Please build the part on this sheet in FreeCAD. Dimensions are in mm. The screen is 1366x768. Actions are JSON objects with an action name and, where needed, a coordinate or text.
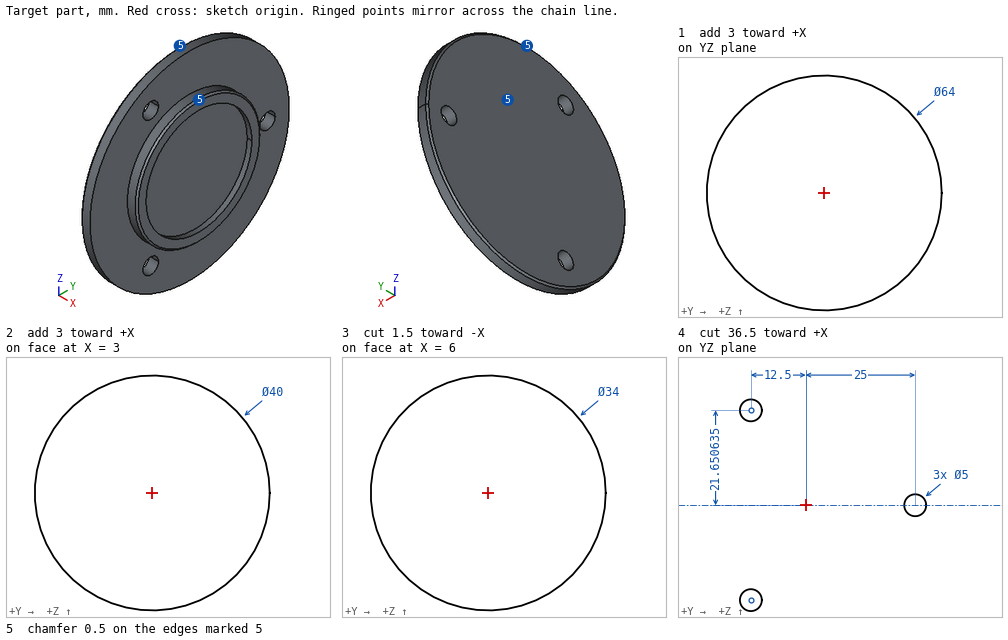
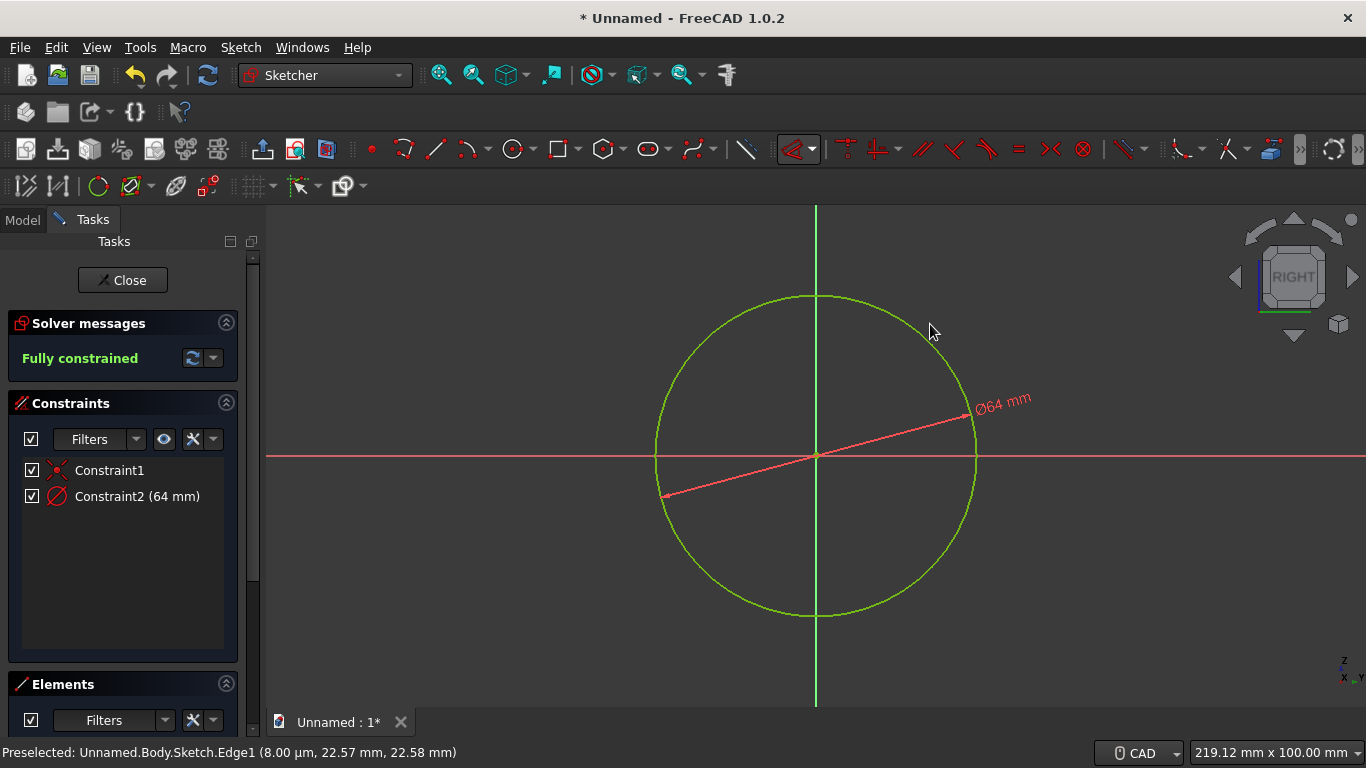
{"action": "left_click", "coordinate": [123, 280]}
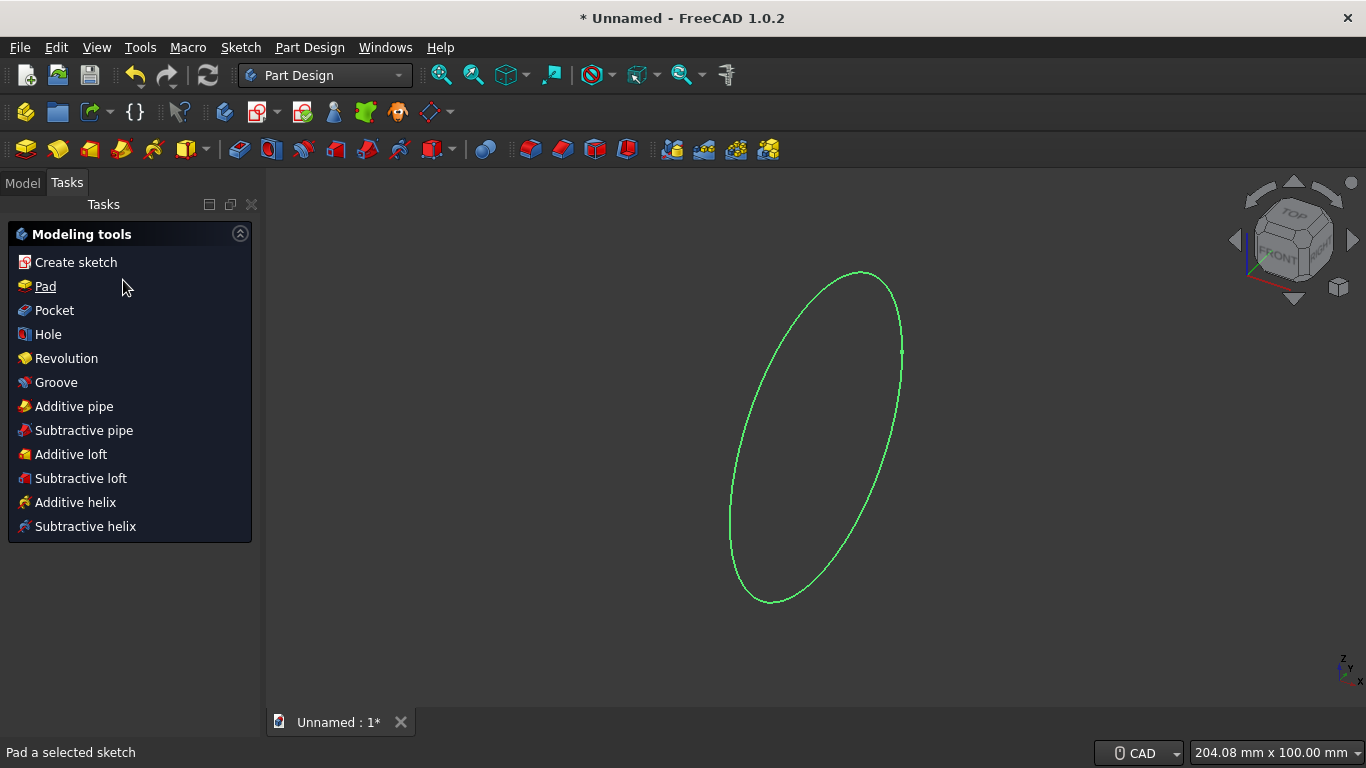
{"action": "left_click", "coordinate": [26, 150]}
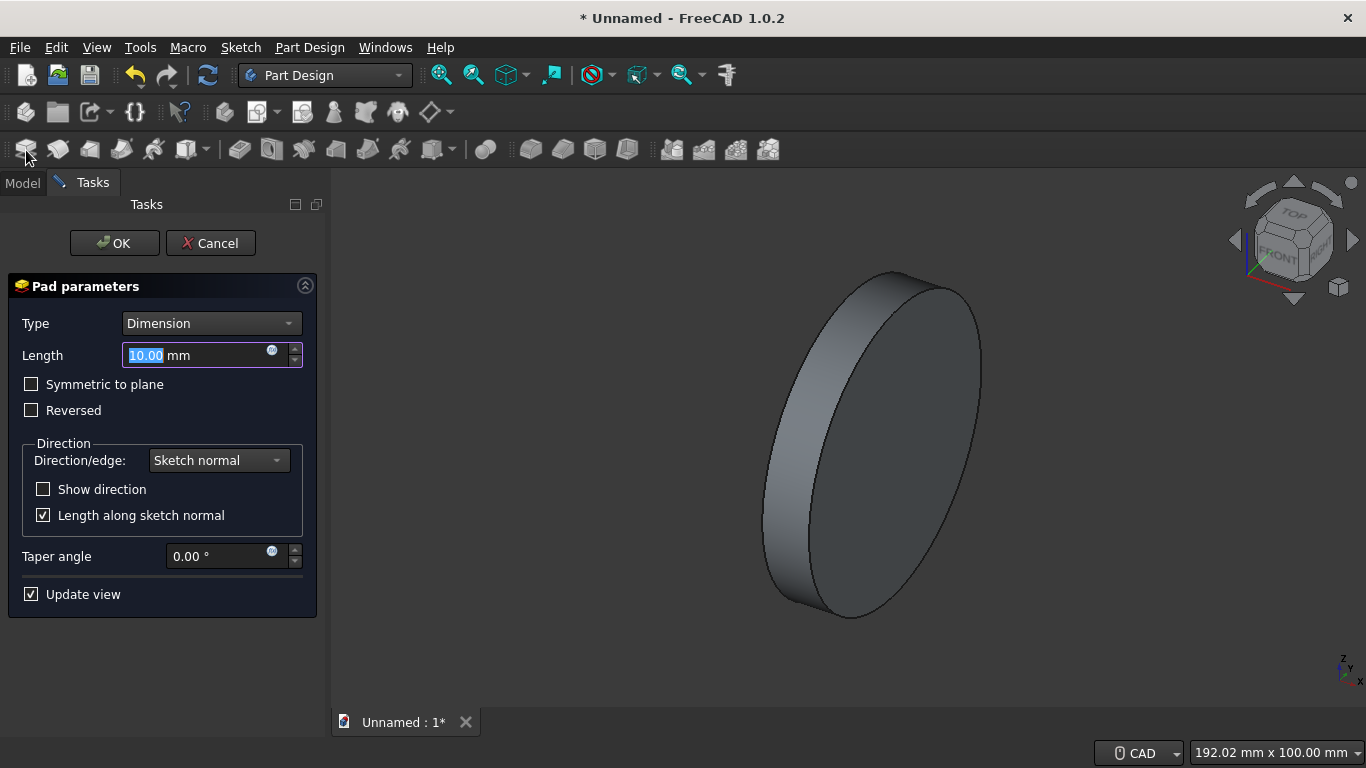
{"action": "type", "text": "3"}
{"action": "key", "text": "Tab"}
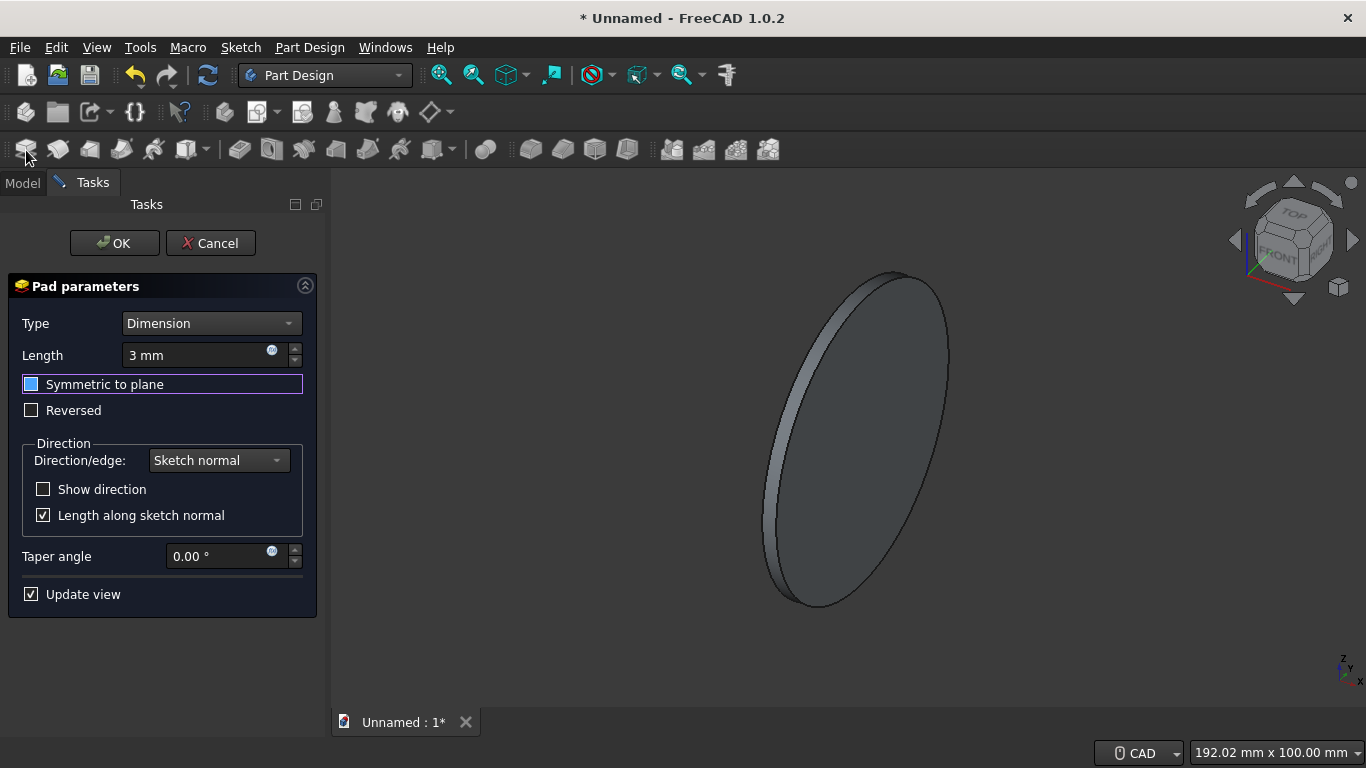
{"action": "left_click", "coordinate": [115, 243]}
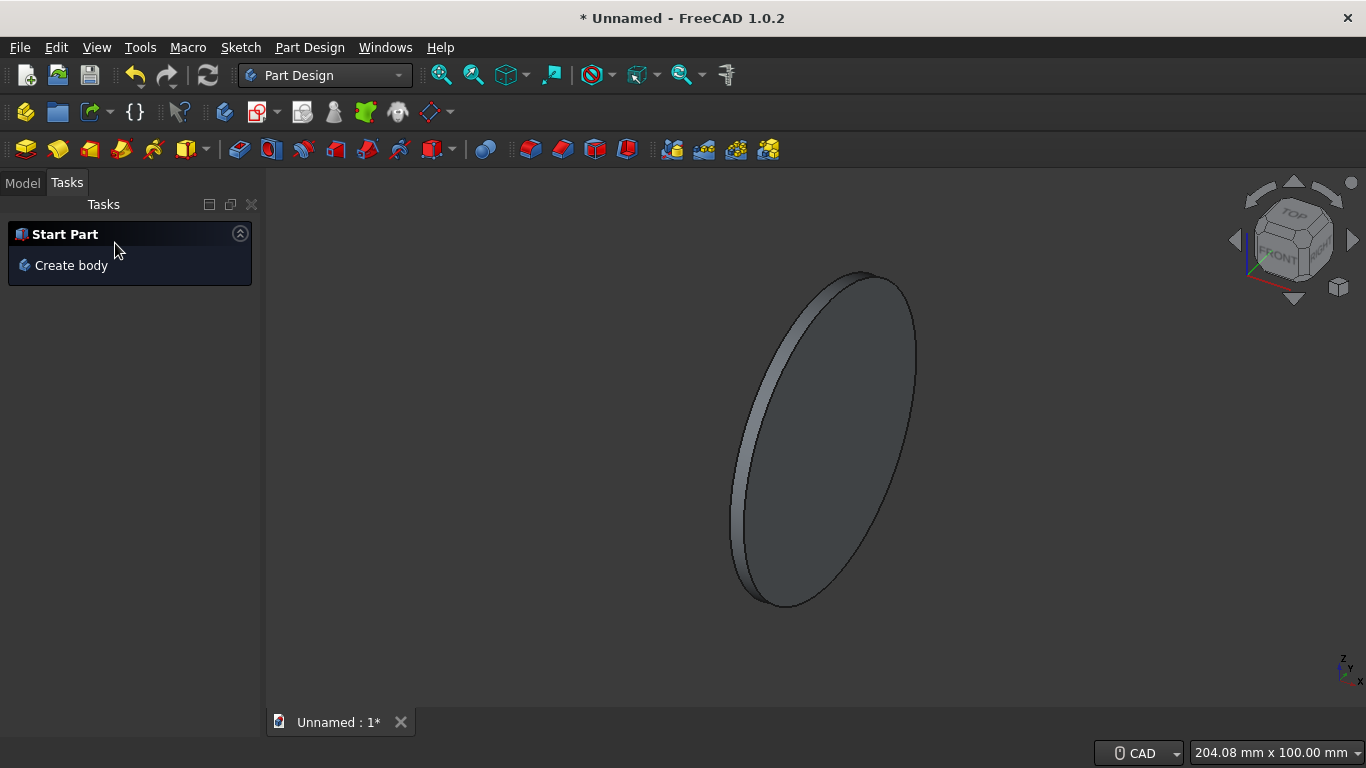
{"action": "left_click", "coordinate": [830, 441]}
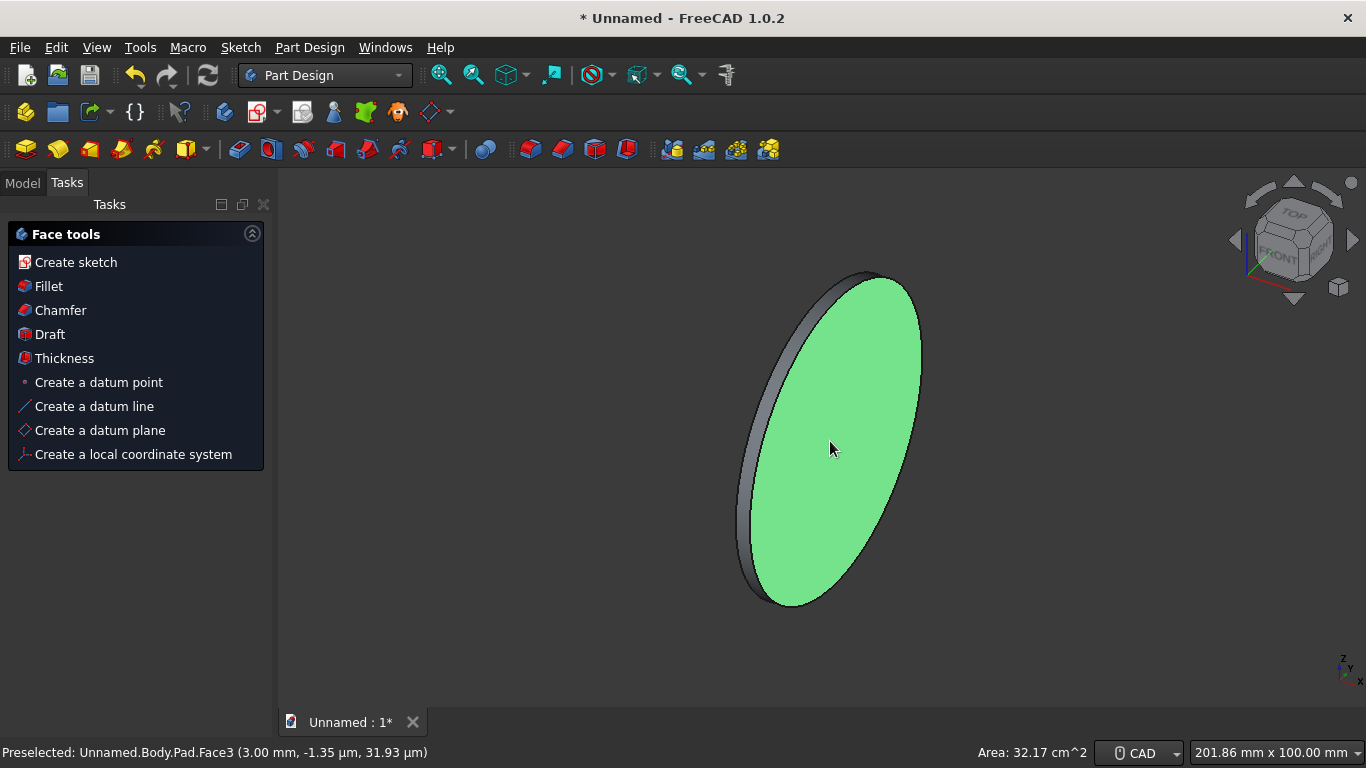
{"action": "left_click", "coordinate": [258, 112]}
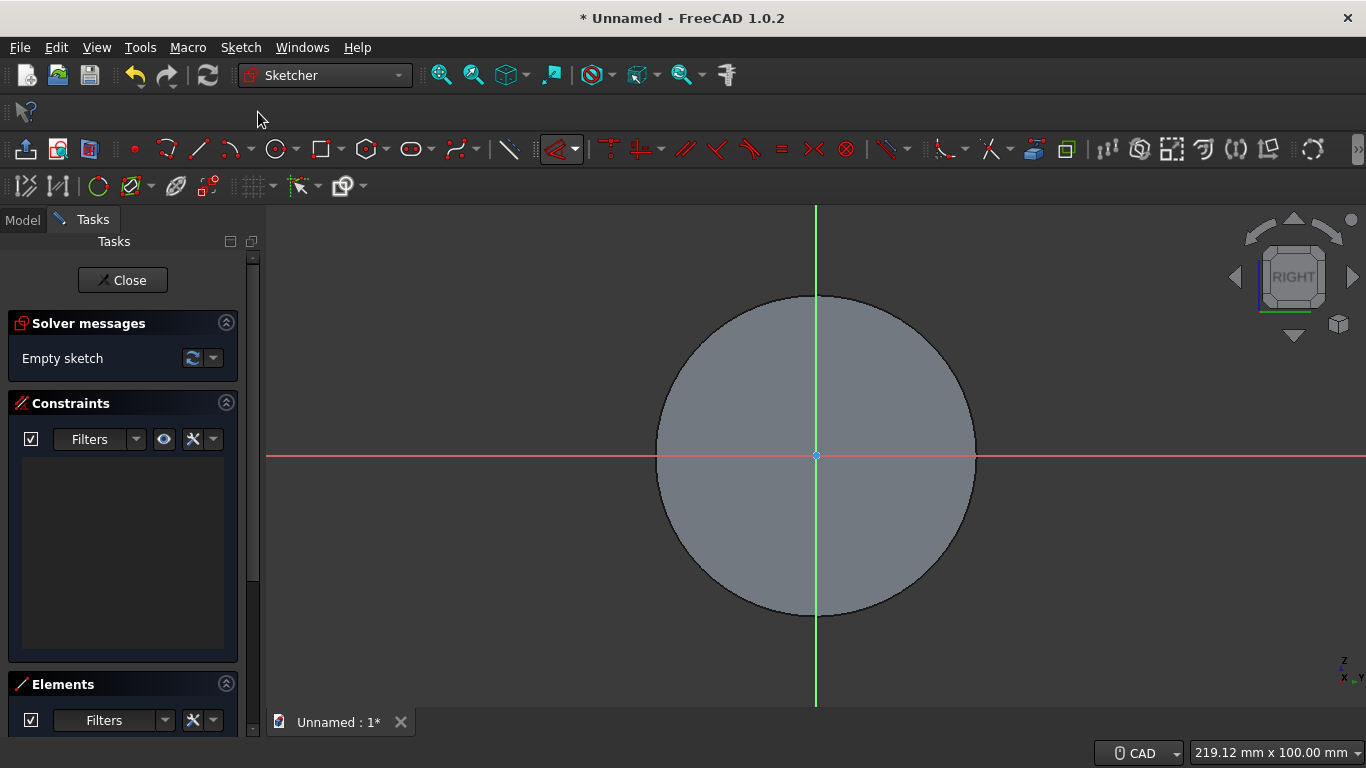
{"action": "scroll", "coordinate": [955, 456], "scroll_direction": "up", "scroll_amount": 2}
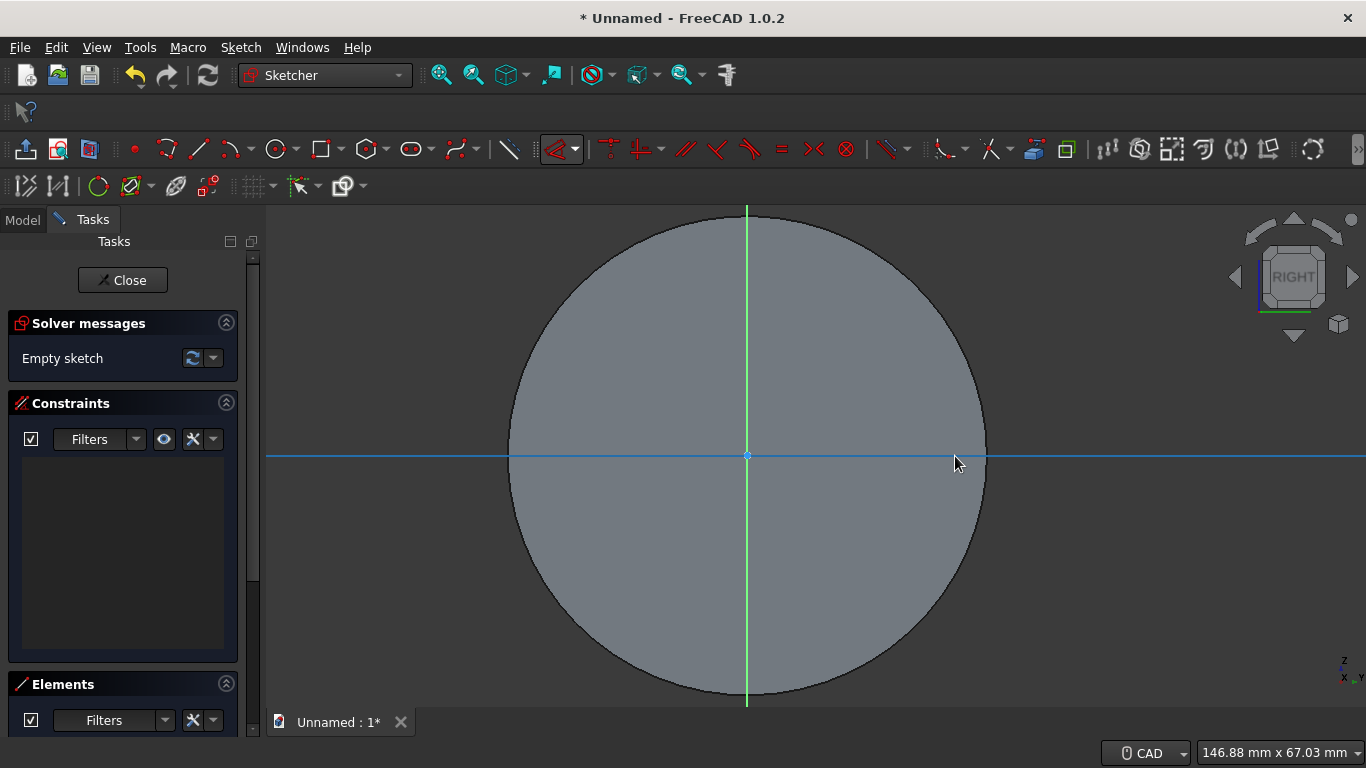
{"action": "left_click", "coordinate": [276, 150]}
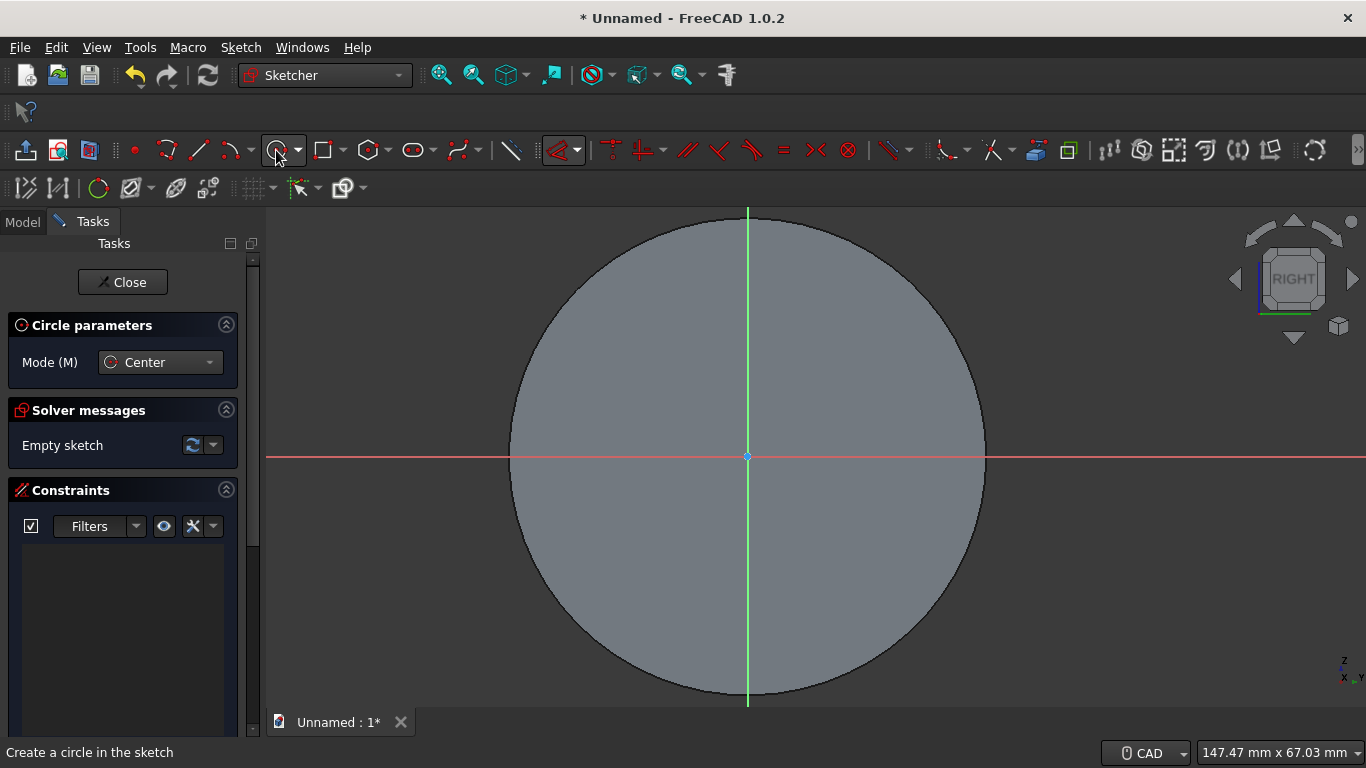
{"action": "left_click", "coordinate": [748, 457]}
{"action": "left_click", "coordinate": [853, 351]}
{"action": "key", "text": "Escape"}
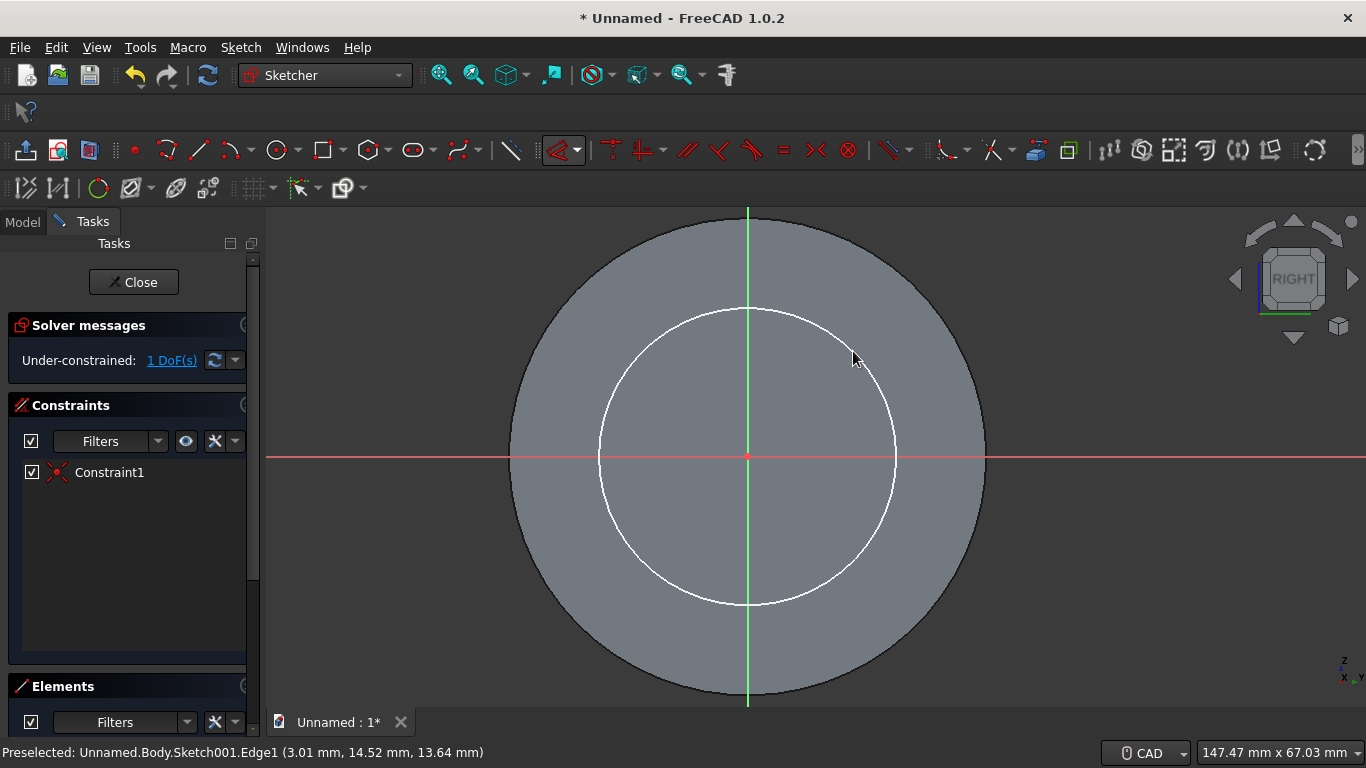
{"action": "left_click", "coordinate": [852, 351]}